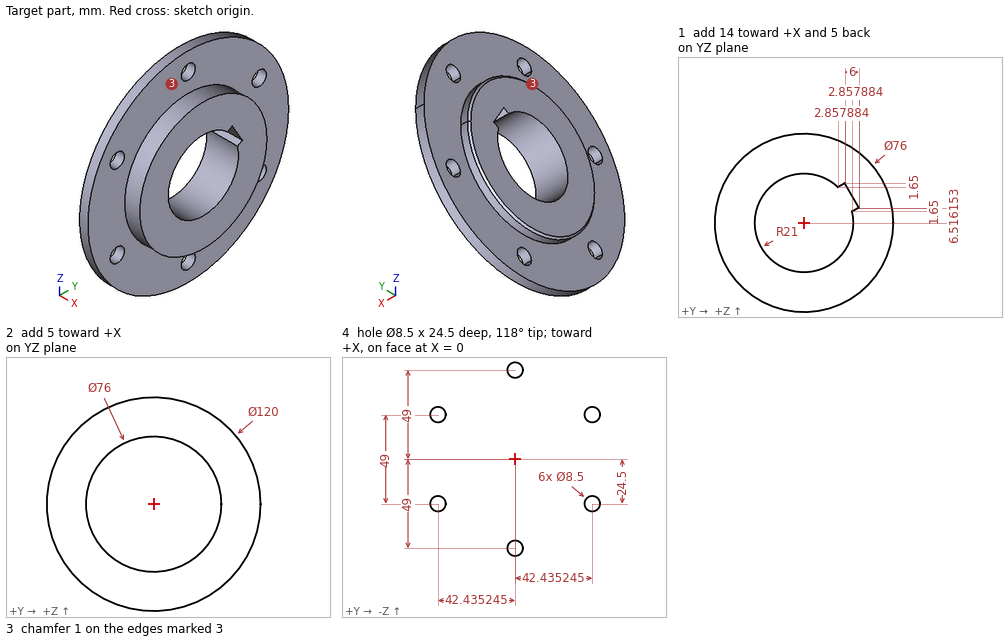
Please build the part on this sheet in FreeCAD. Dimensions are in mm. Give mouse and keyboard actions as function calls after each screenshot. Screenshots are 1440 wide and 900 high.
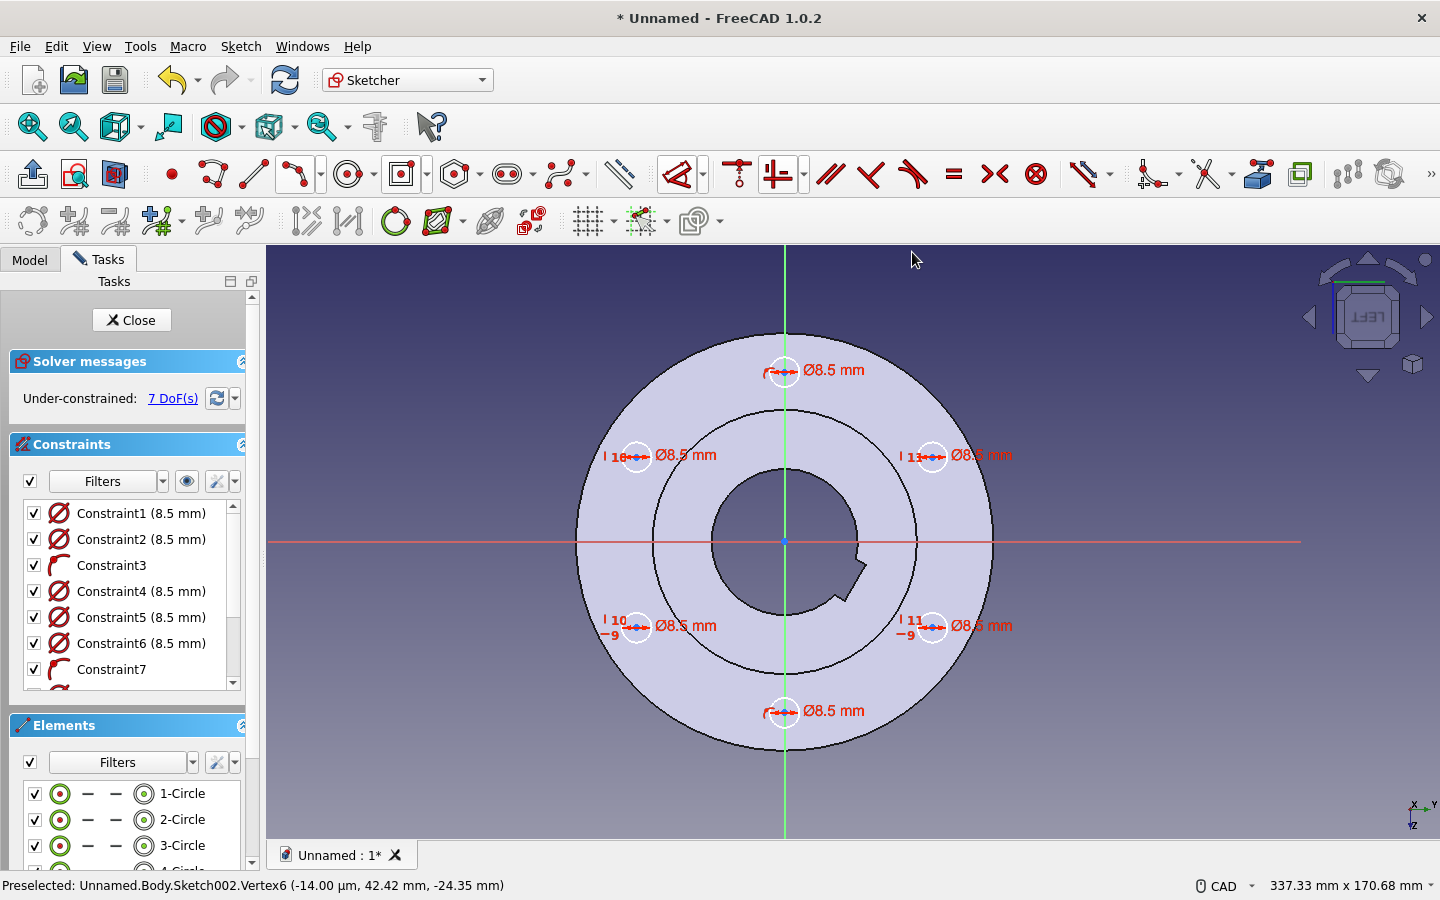
click(637, 457)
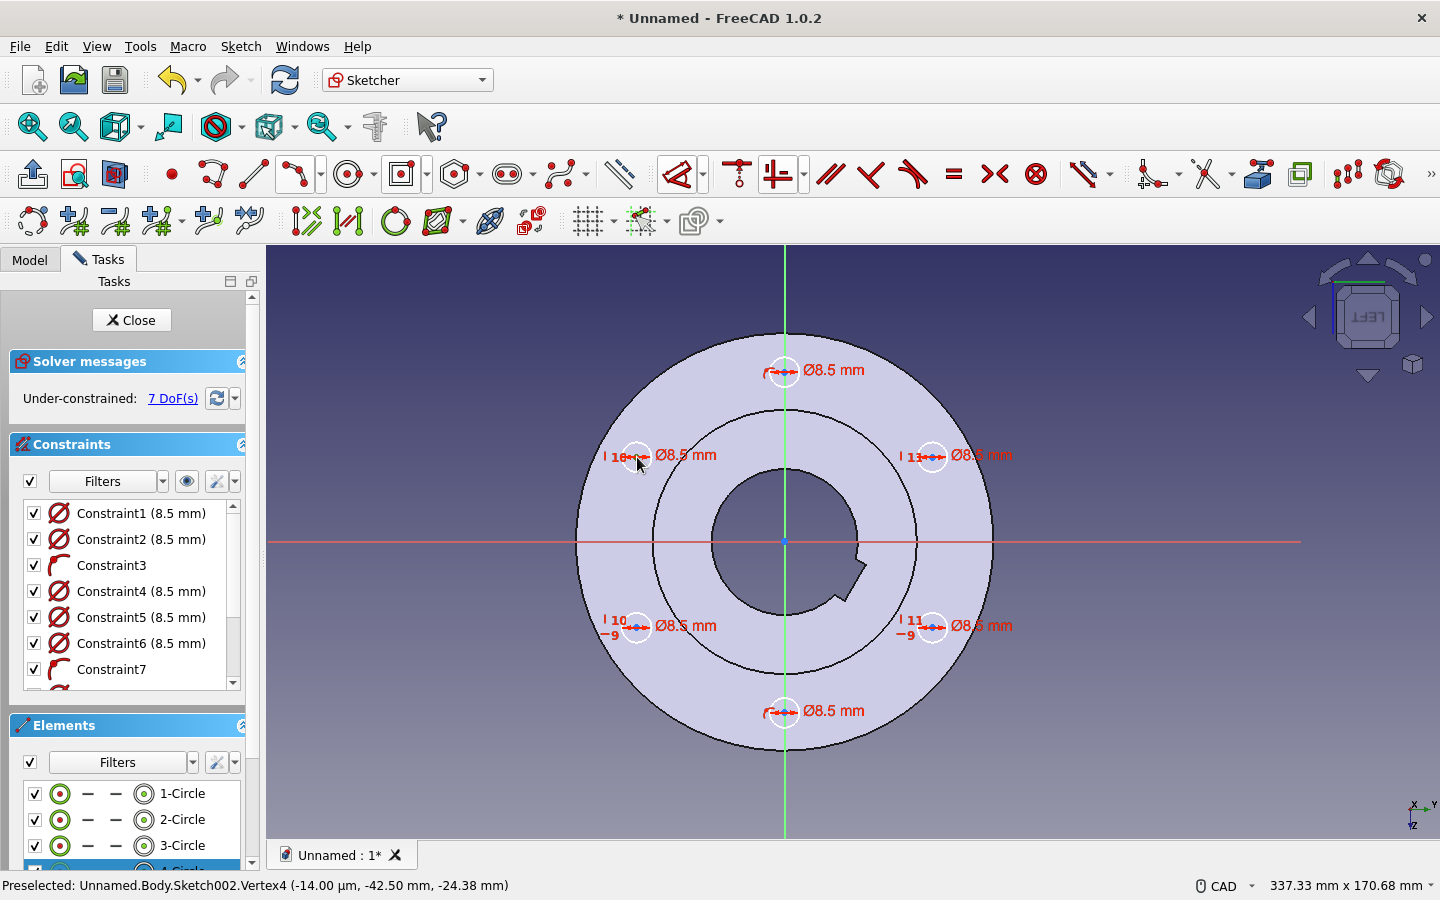
click(933, 457)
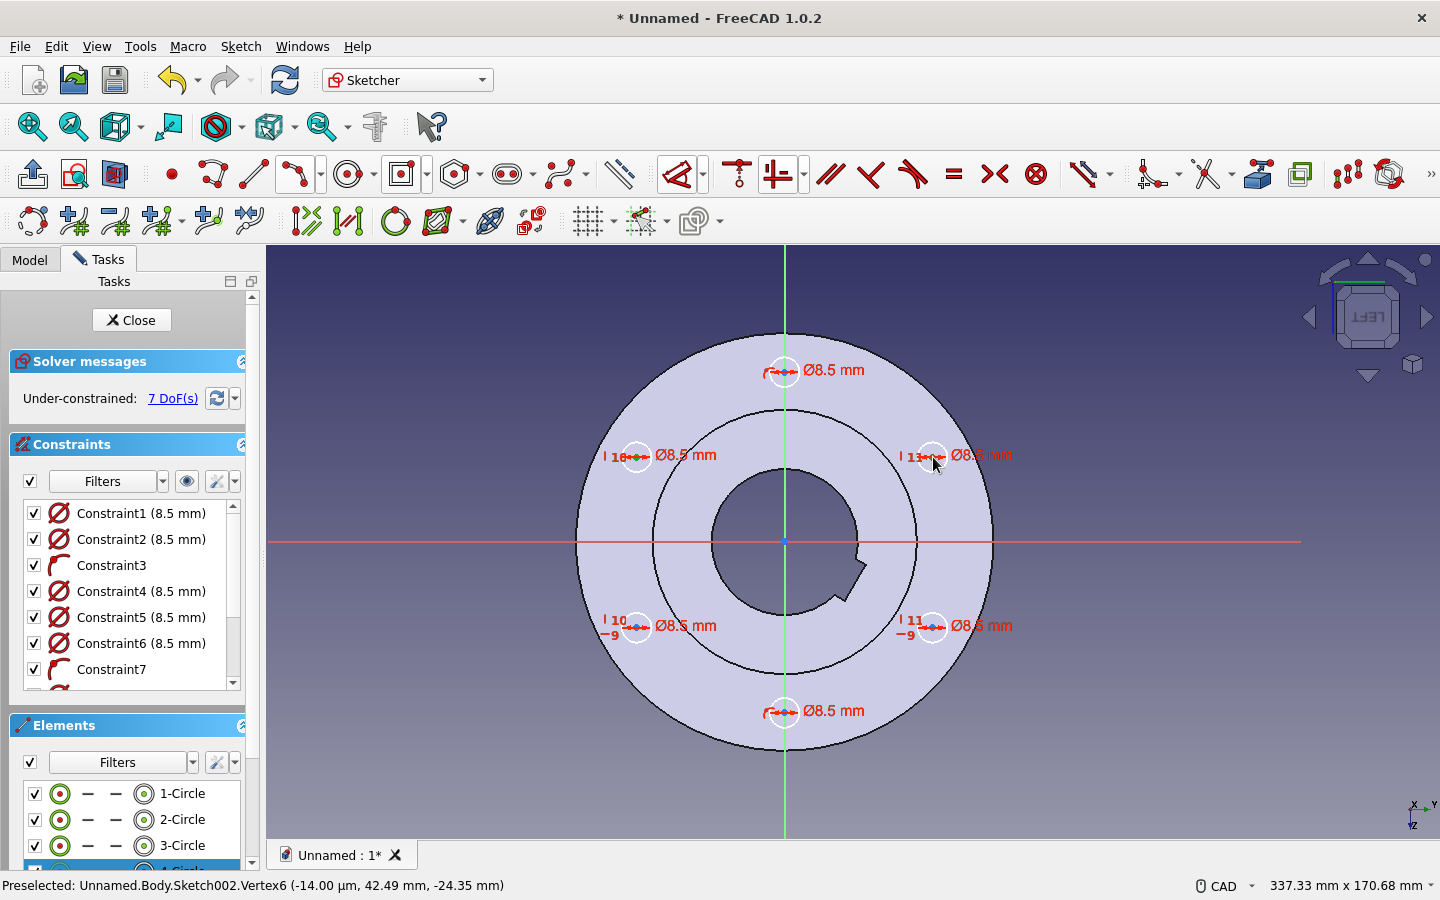
key(h)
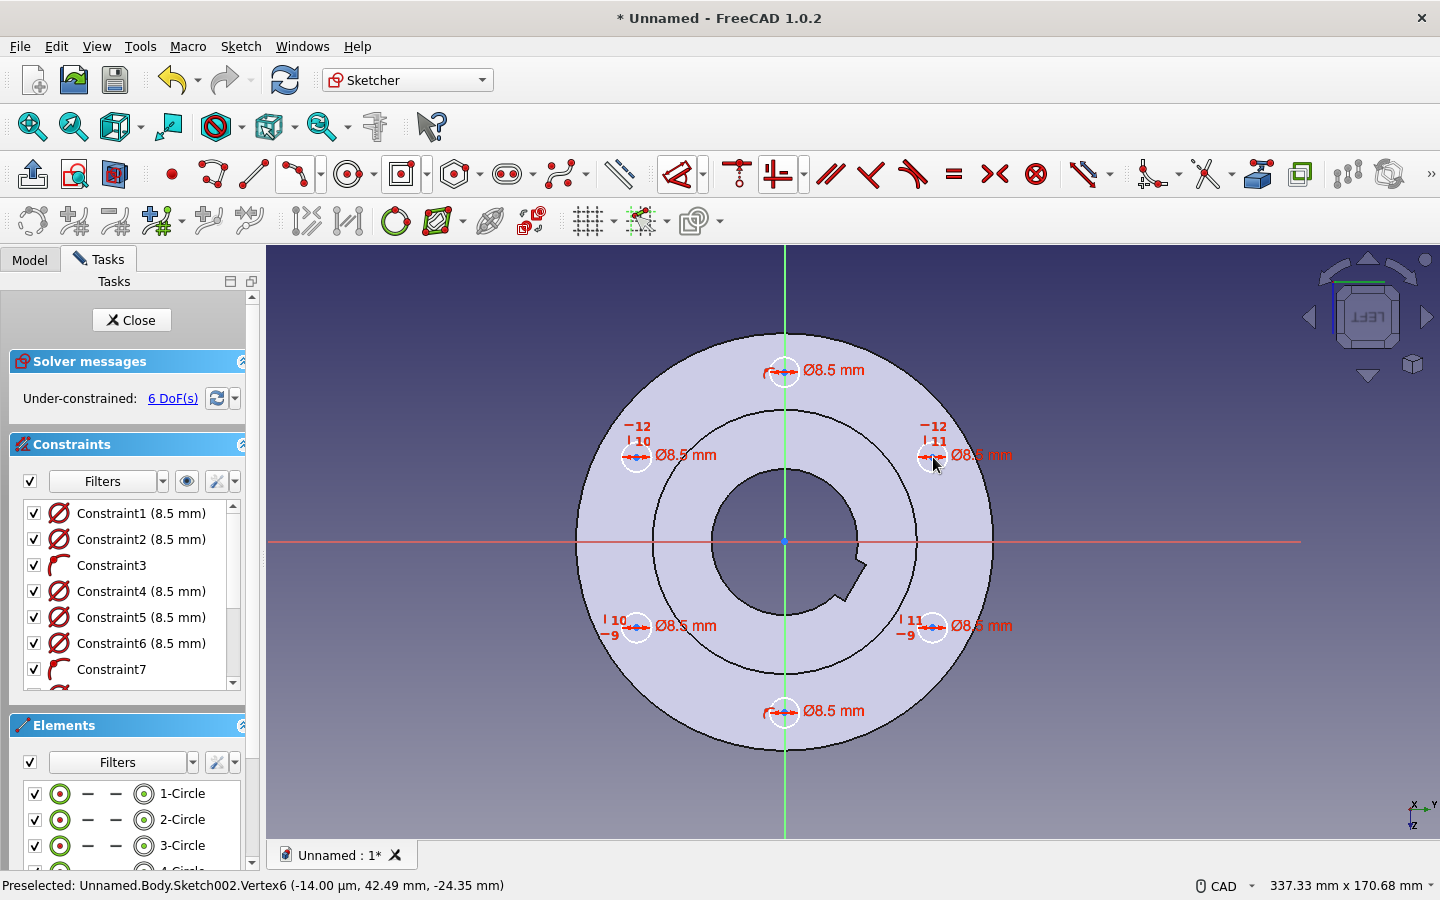
key(d)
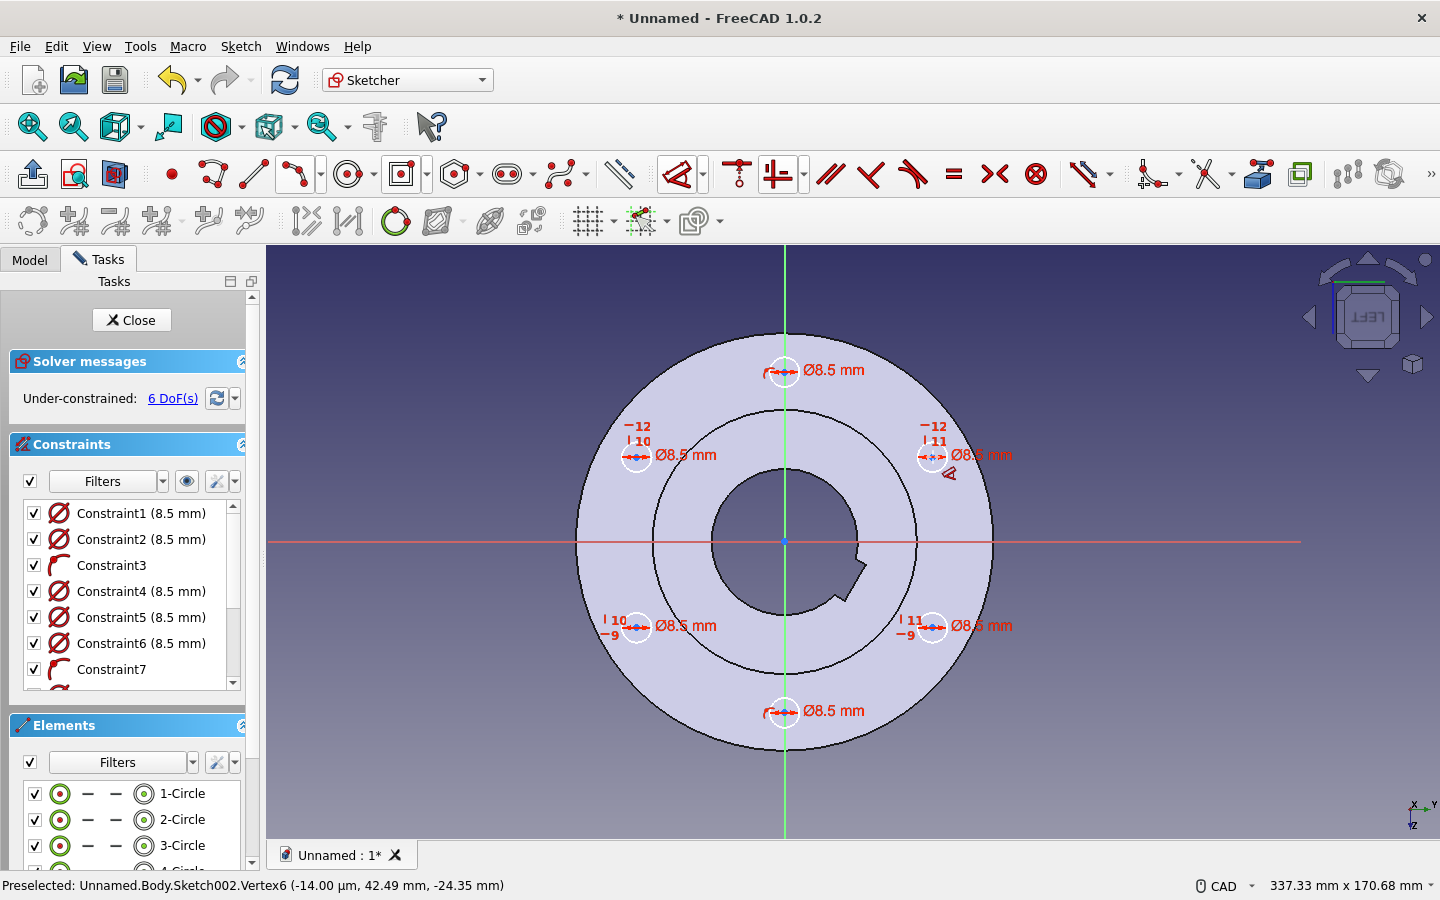
click(785, 713)
click(819, 627)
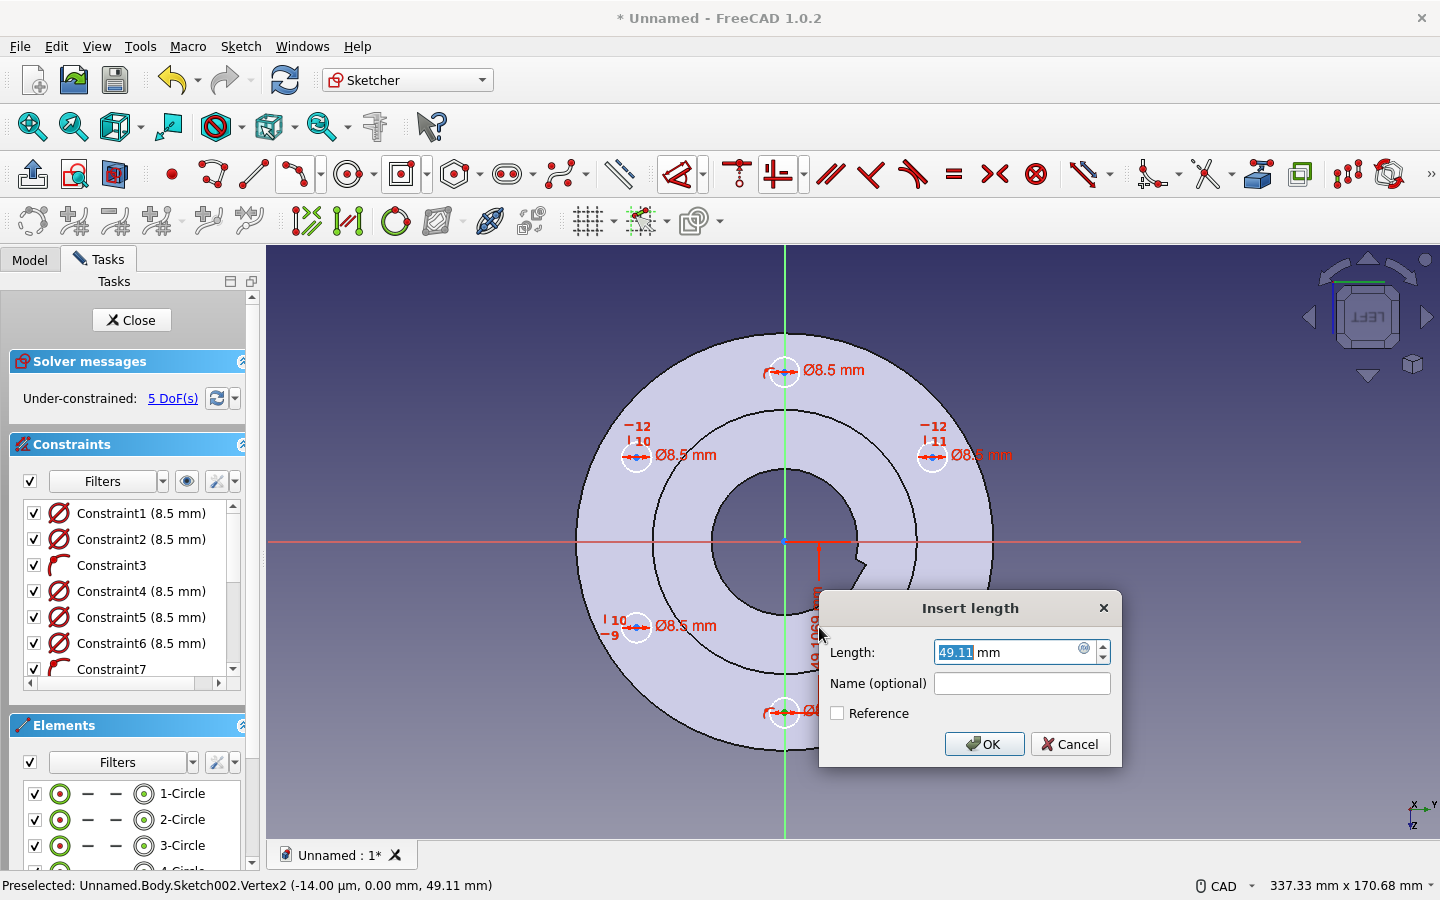
text(49)
key(Return)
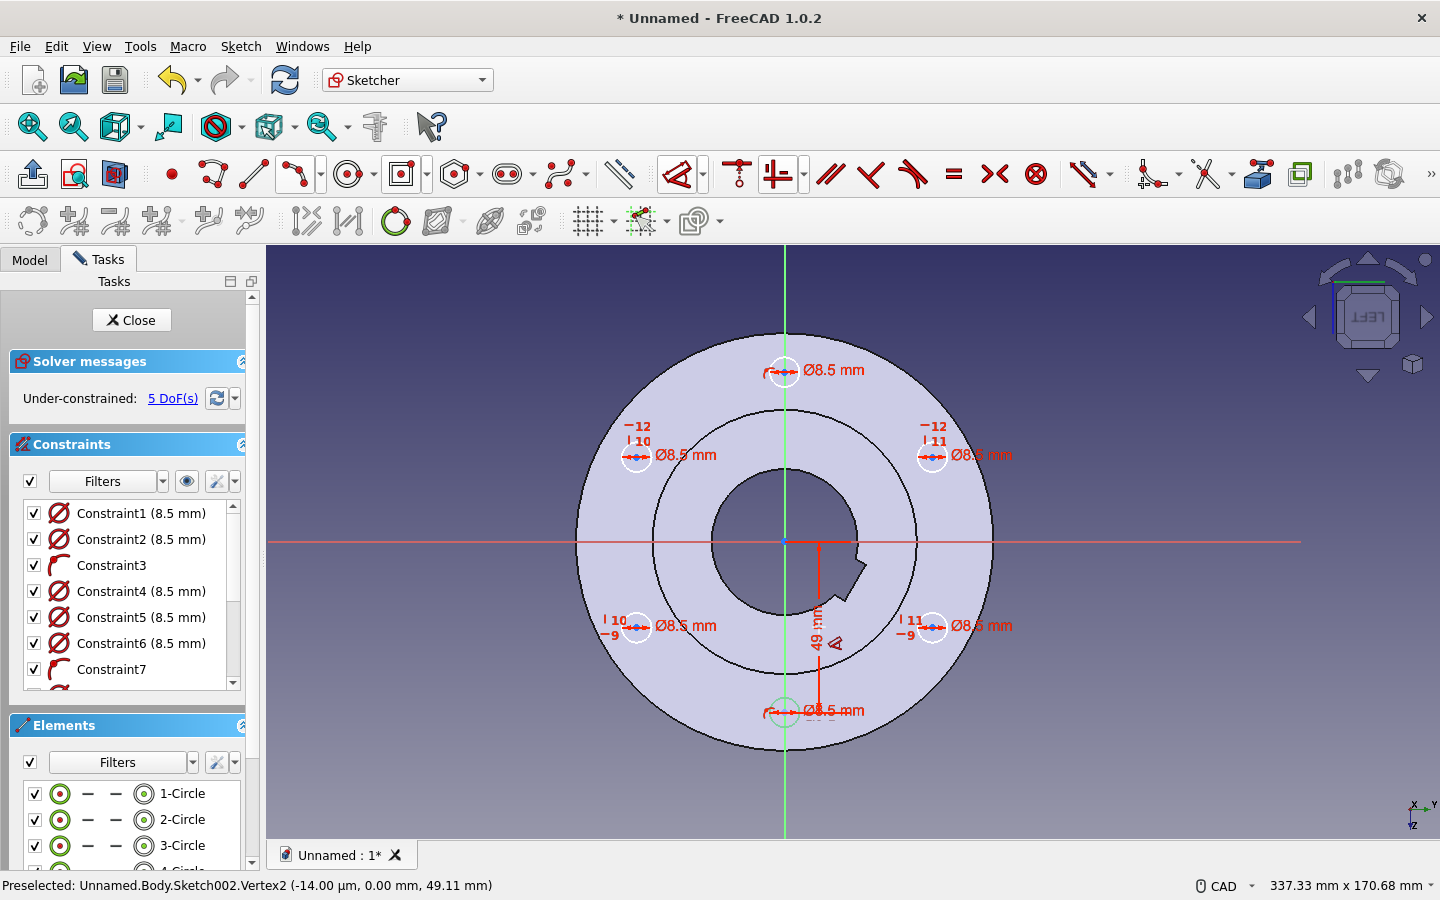
click(785, 372)
click(819, 457)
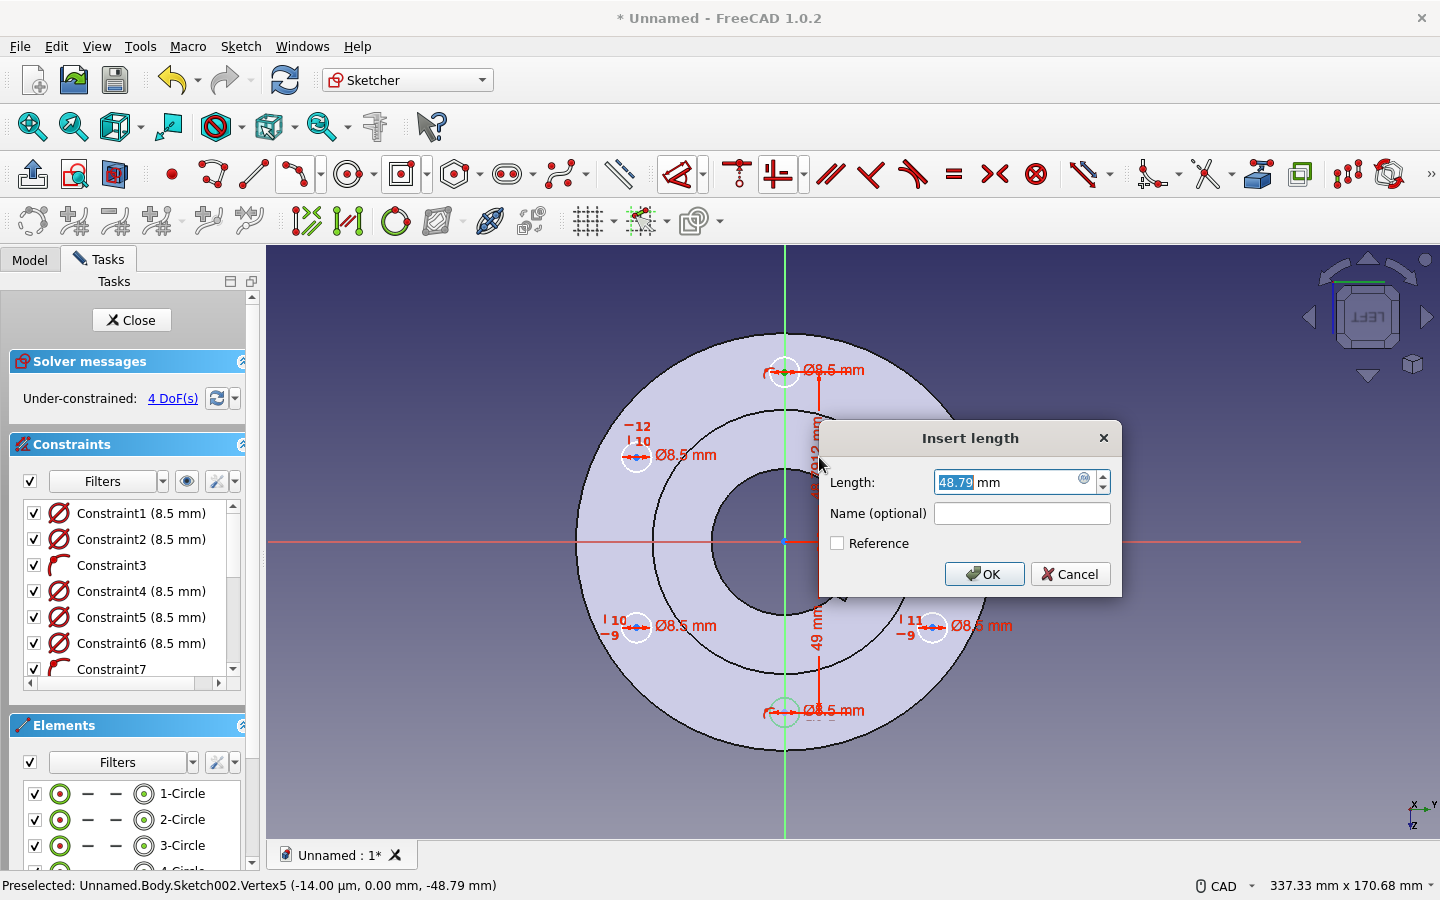
text(49)
key(Return)